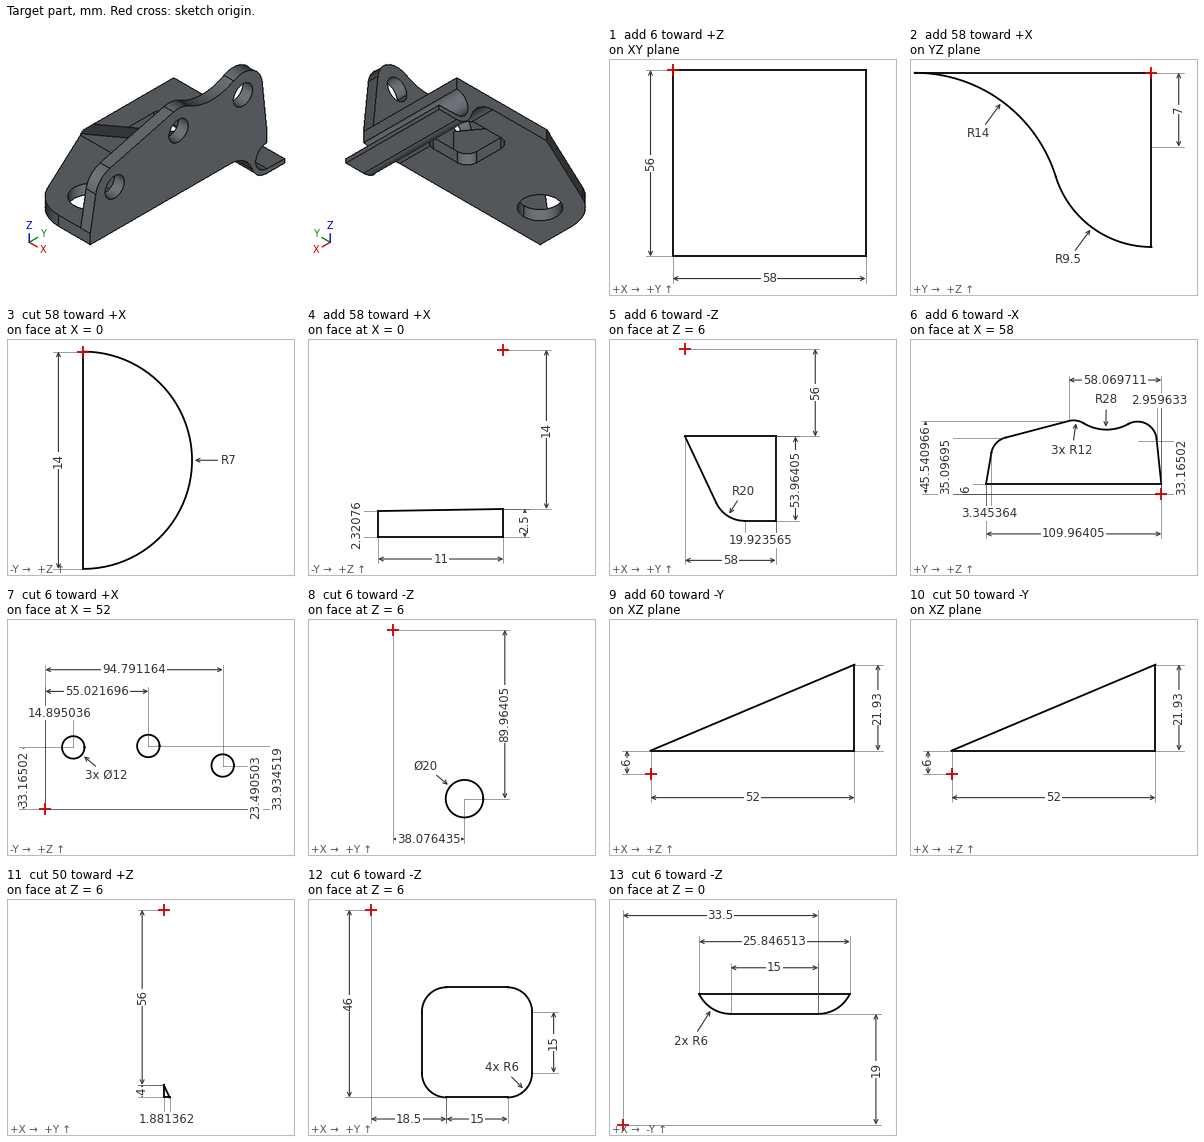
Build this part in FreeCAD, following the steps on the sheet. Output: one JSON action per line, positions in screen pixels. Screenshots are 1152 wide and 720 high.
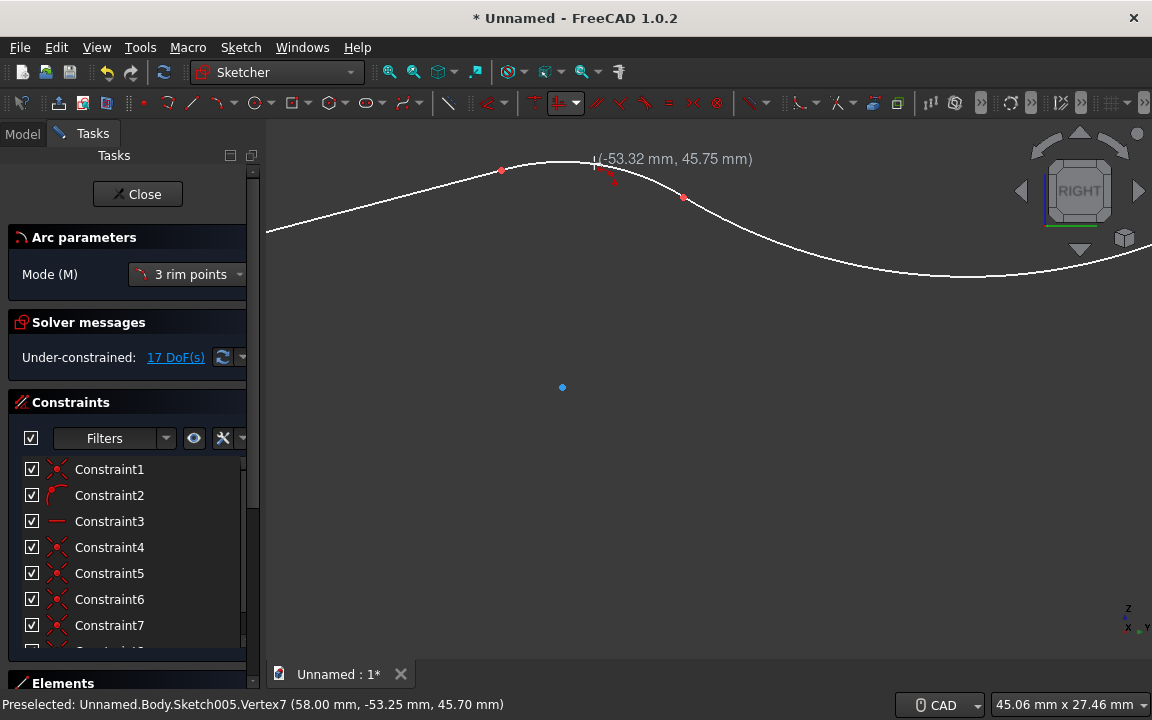
{"action": "scroll", "coordinate": [666, 316], "scroll_direction": "down", "scroll_amount": 7}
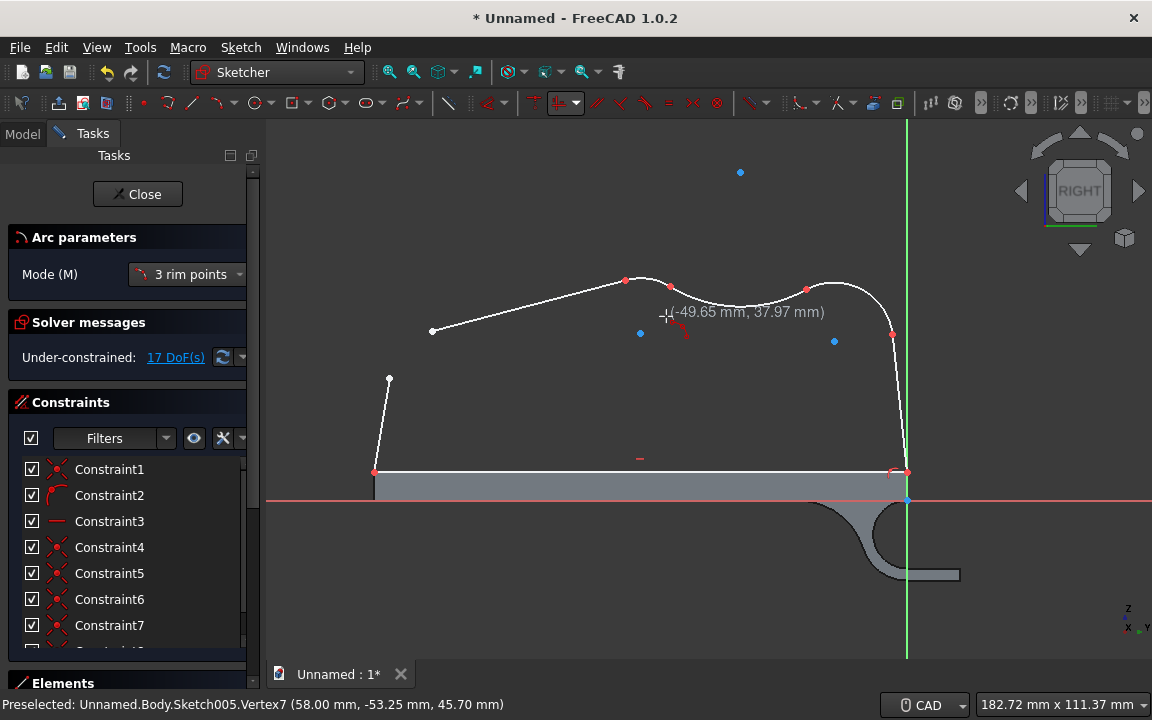
{"action": "left_click", "coordinate": [432, 331]}
{"action": "left_click", "coordinate": [390, 378]}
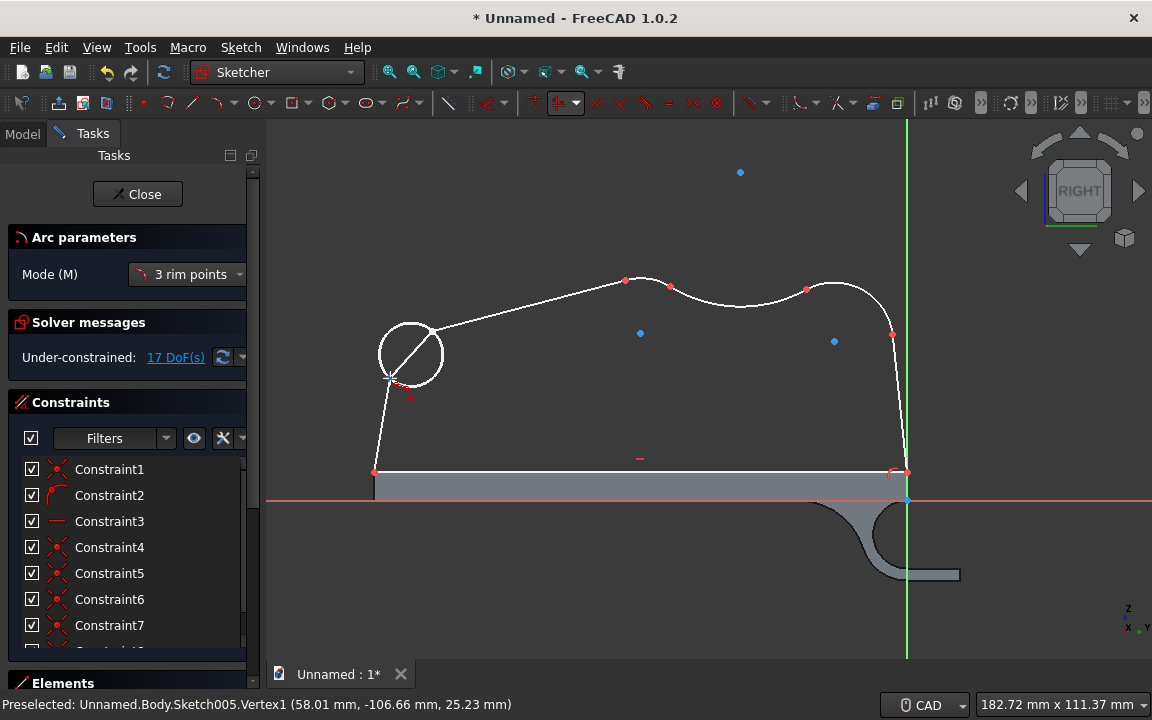
{"action": "scroll", "coordinate": [405, 347], "scroll_direction": "up", "scroll_amount": 3}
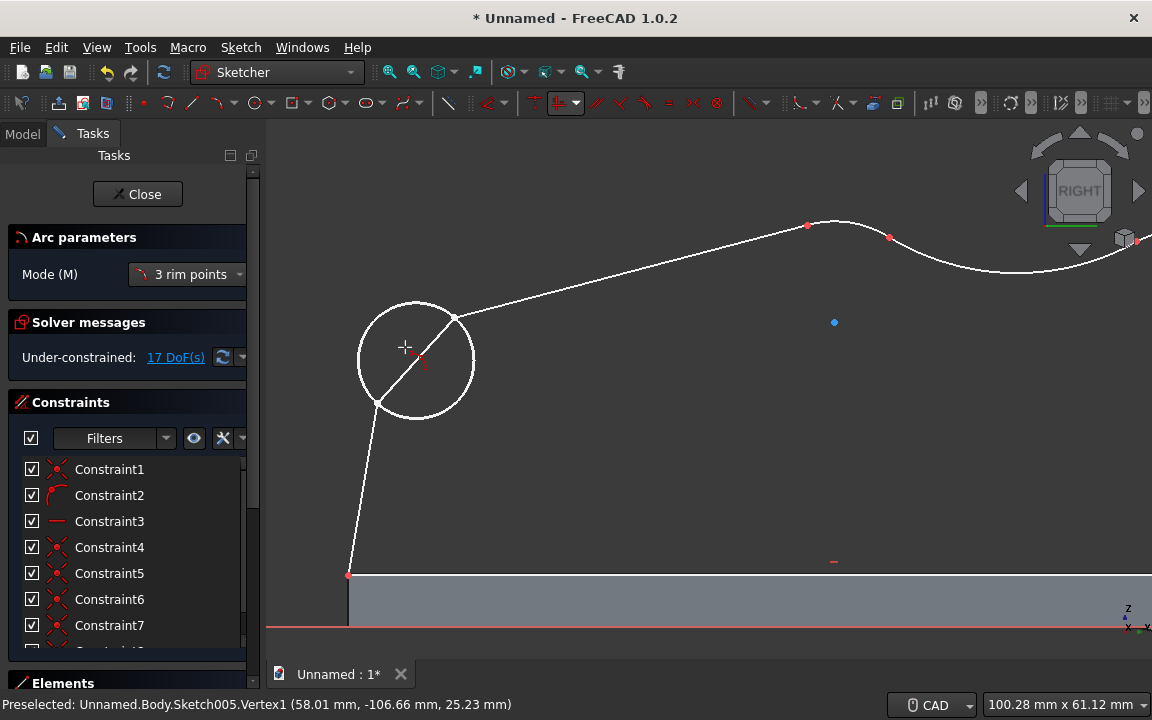
{"action": "left_click", "coordinate": [404, 347]}
{"action": "key", "text": "Escape"}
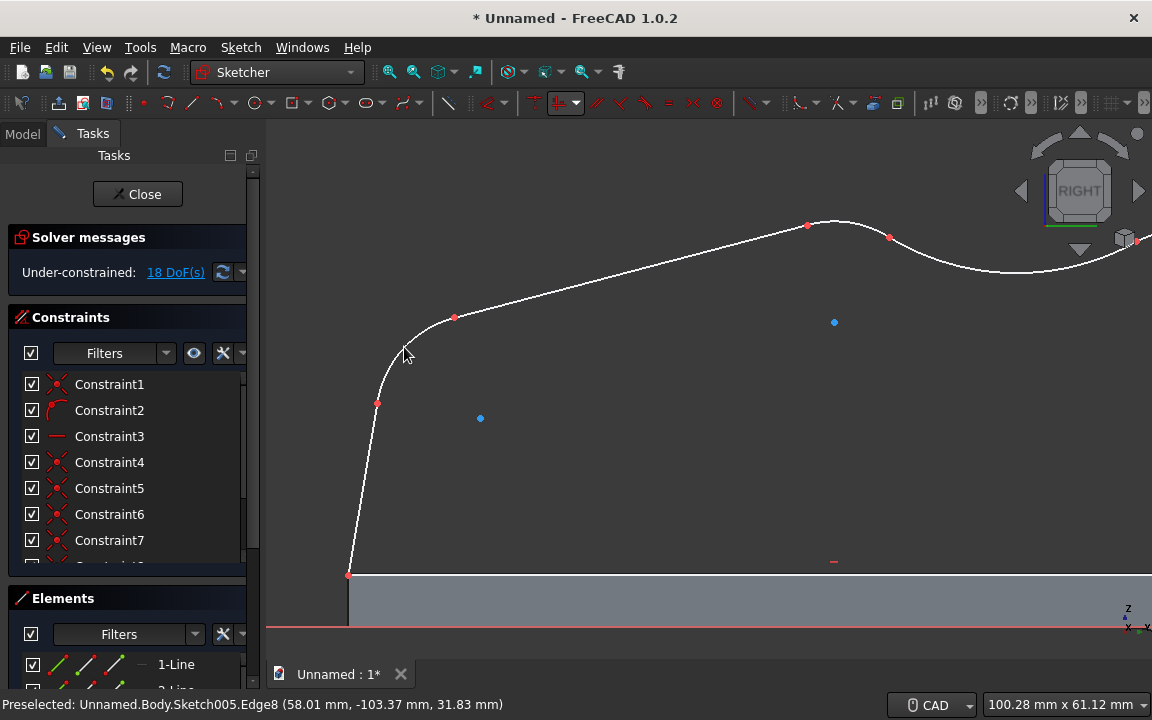
{"action": "left_click", "coordinate": [369, 455]}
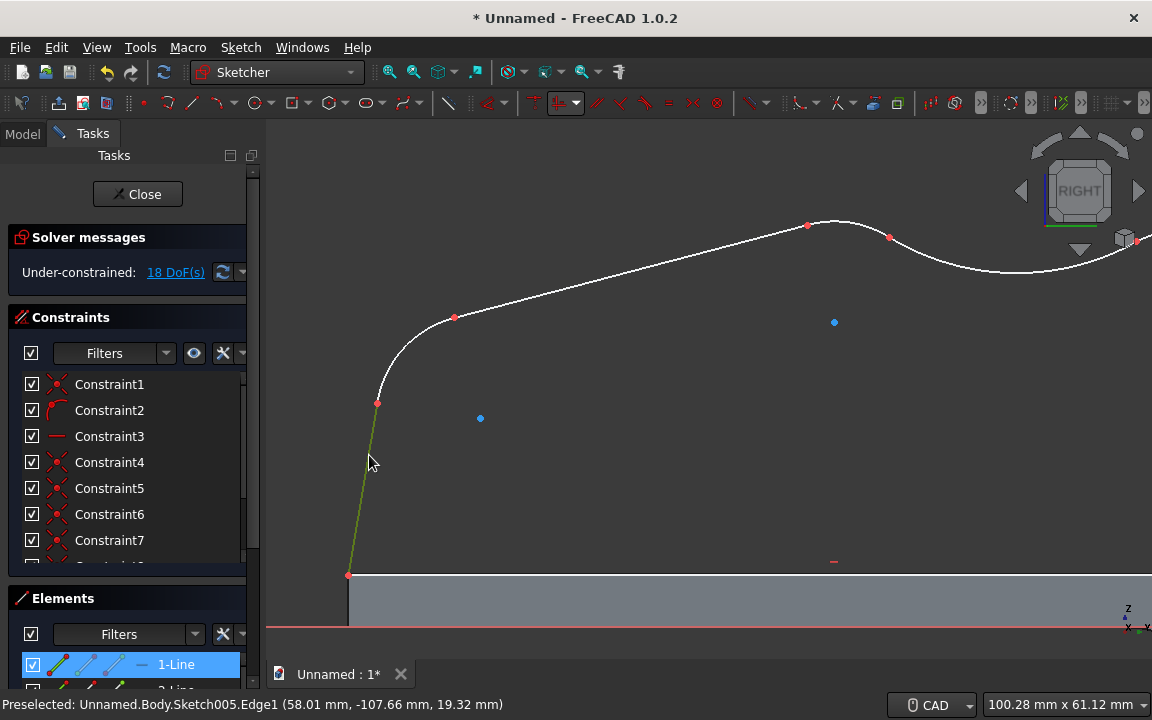
{"action": "left_click", "coordinate": [422, 333]}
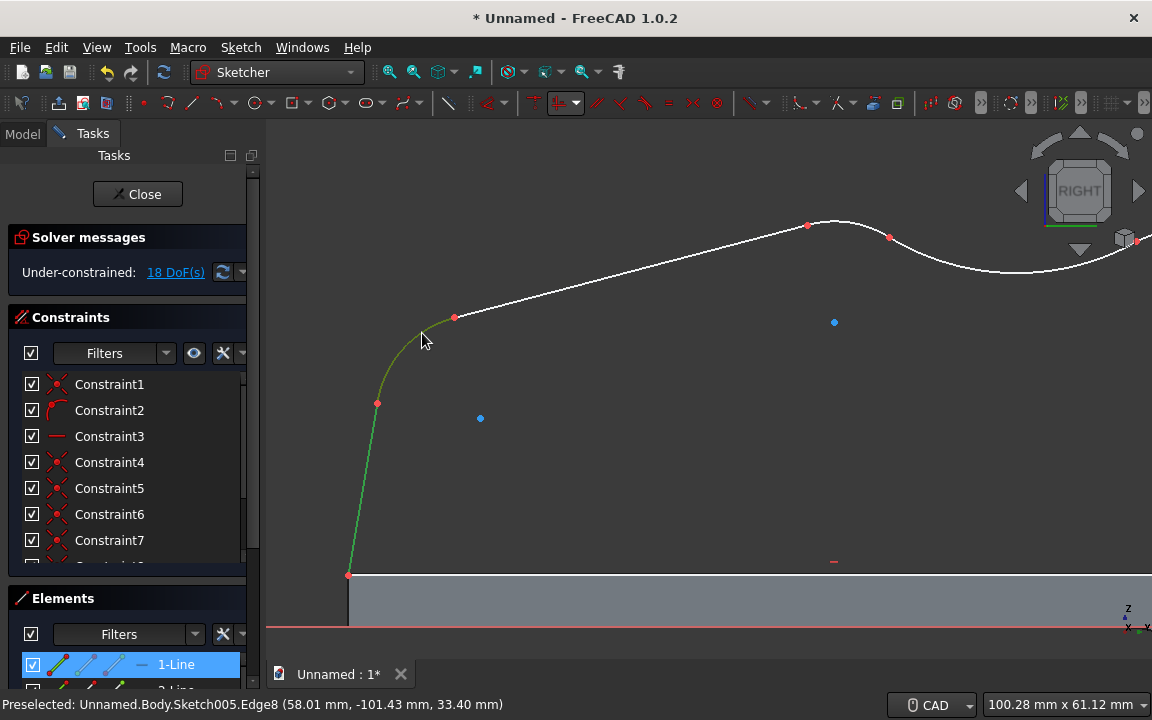
{"action": "key", "text": "t"}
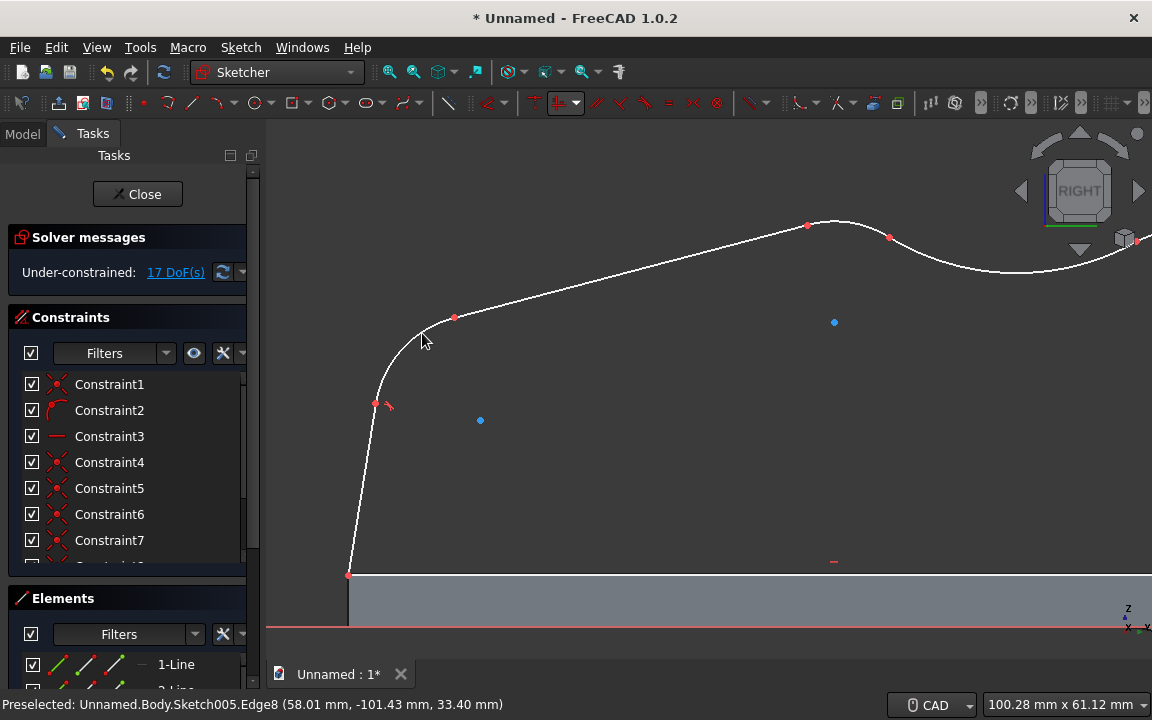
{"action": "scroll", "coordinate": [405, 346], "scroll_direction": "down", "scroll_amount": 3}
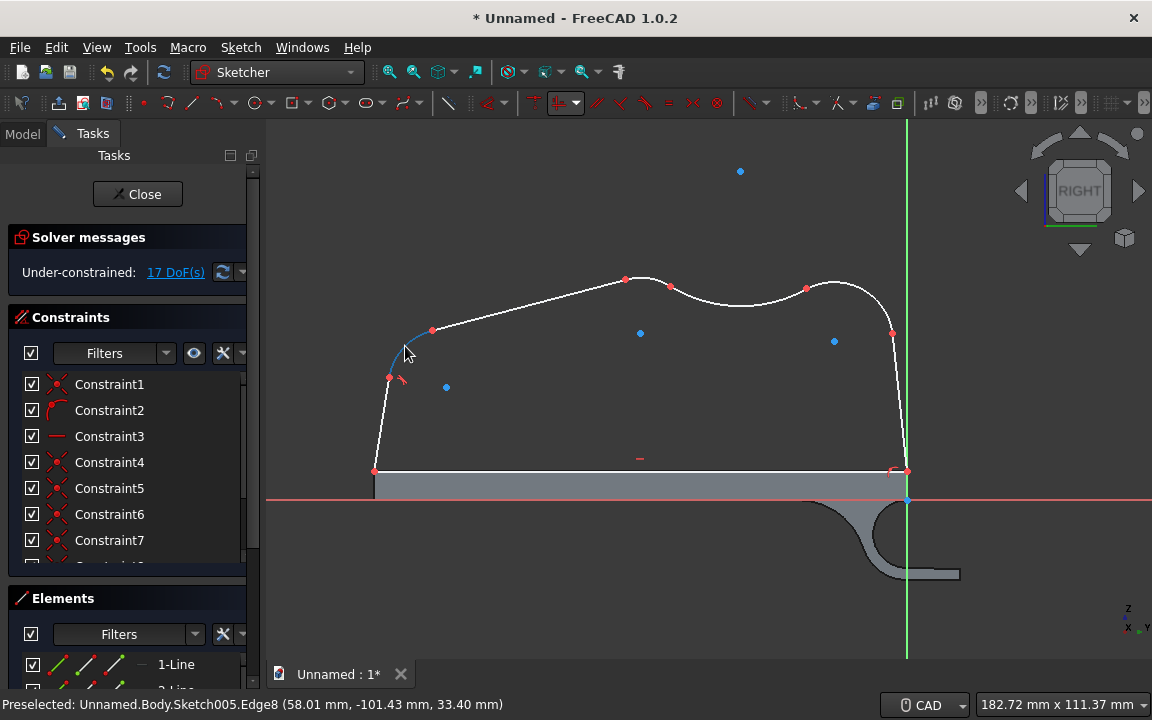
{"action": "scroll", "coordinate": [897, 375], "scroll_direction": "up", "scroll_amount": 2}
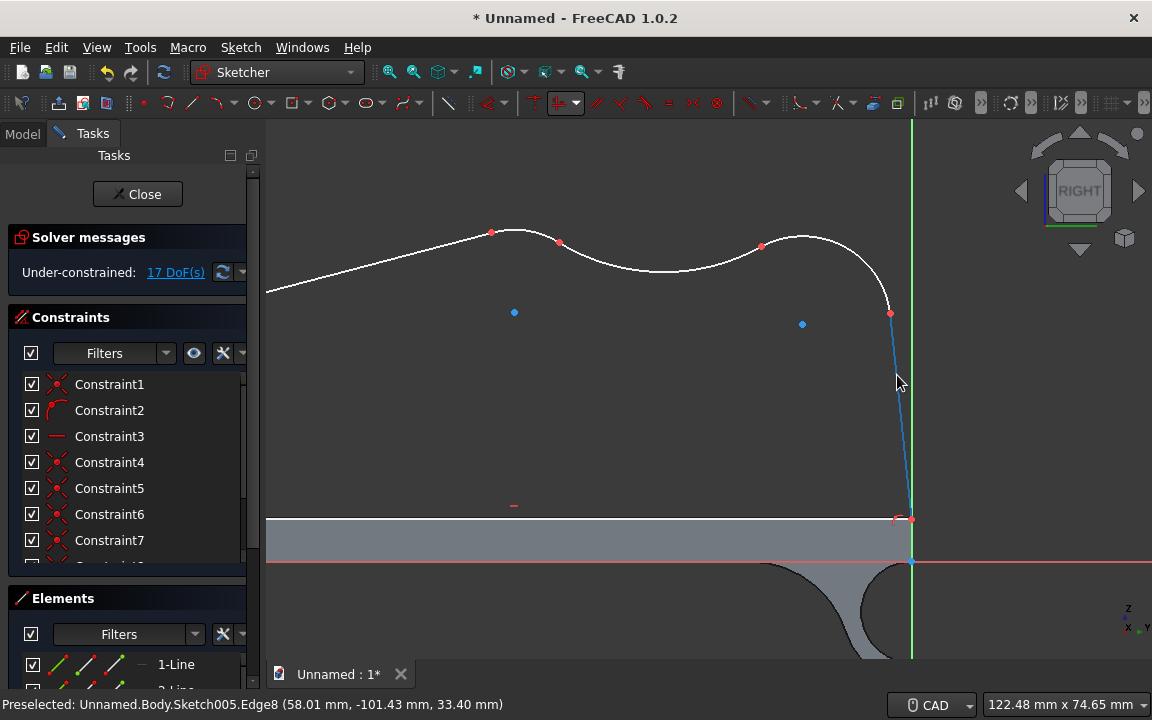
{"action": "left_click", "coordinate": [897, 375]}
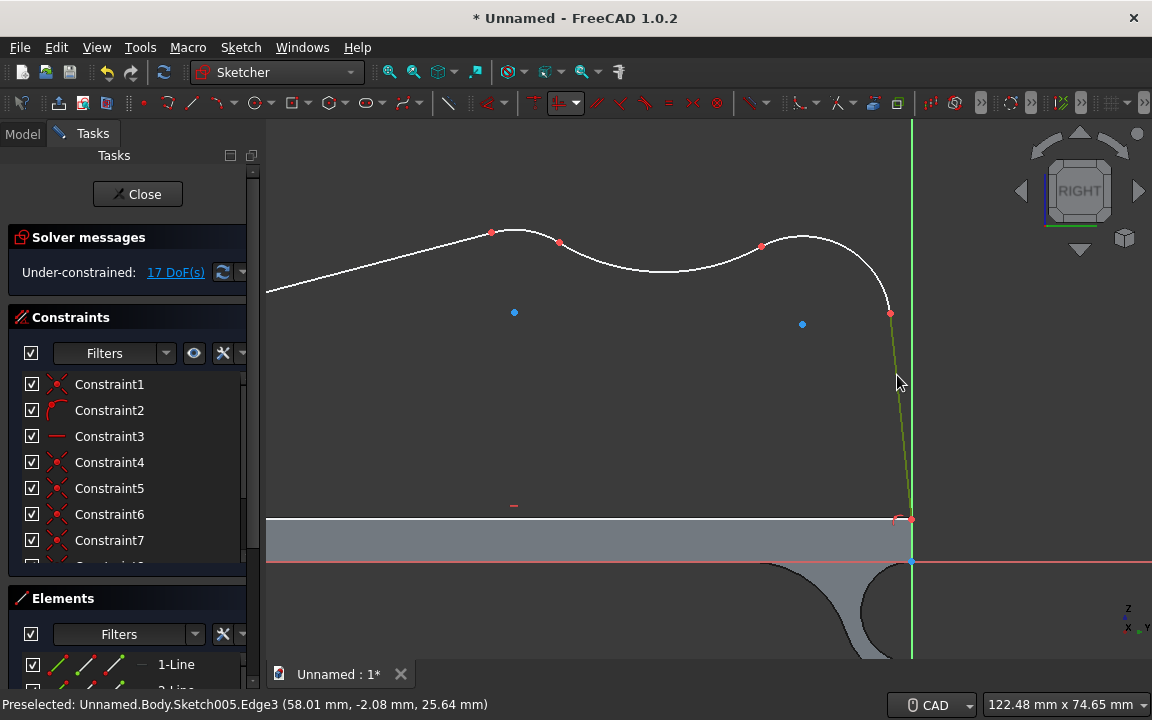
{"action": "left_click", "coordinate": [870, 267]}